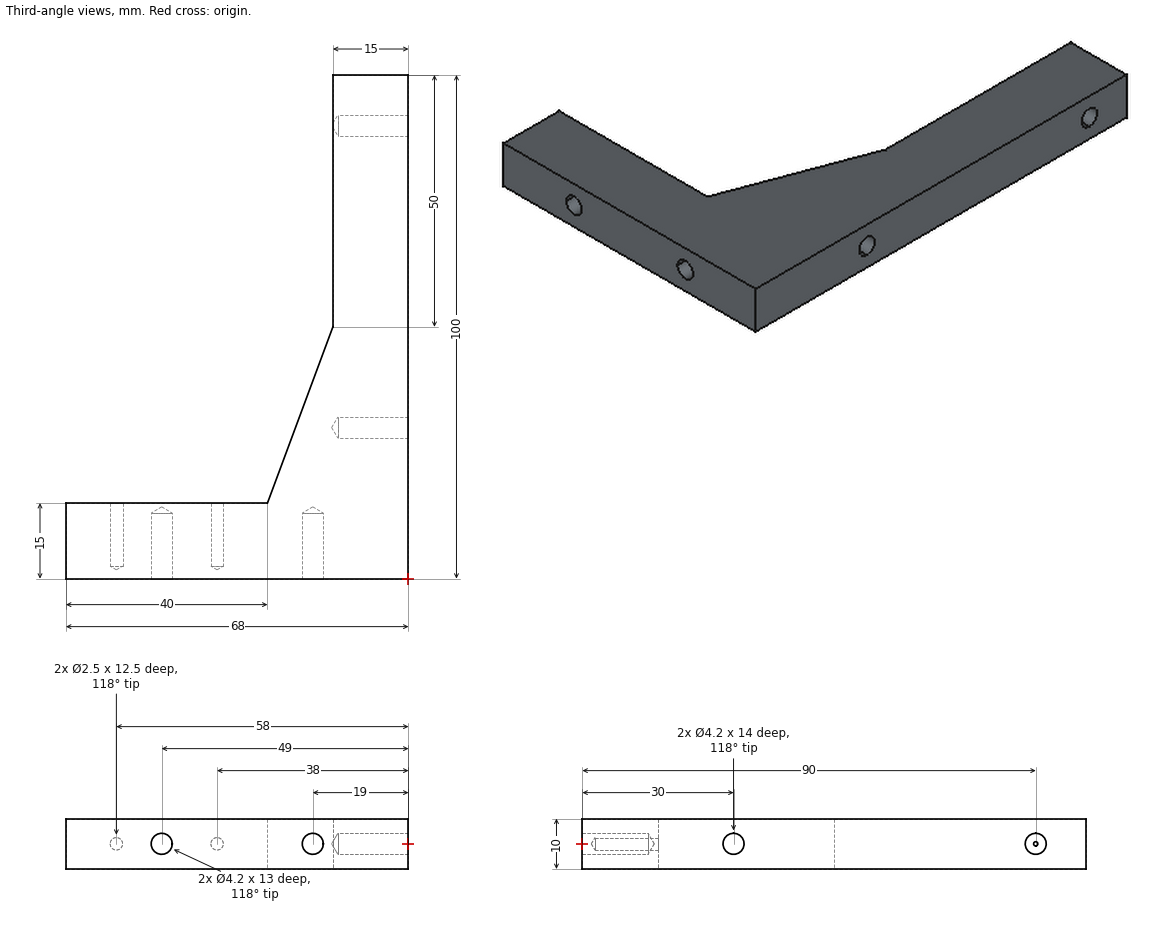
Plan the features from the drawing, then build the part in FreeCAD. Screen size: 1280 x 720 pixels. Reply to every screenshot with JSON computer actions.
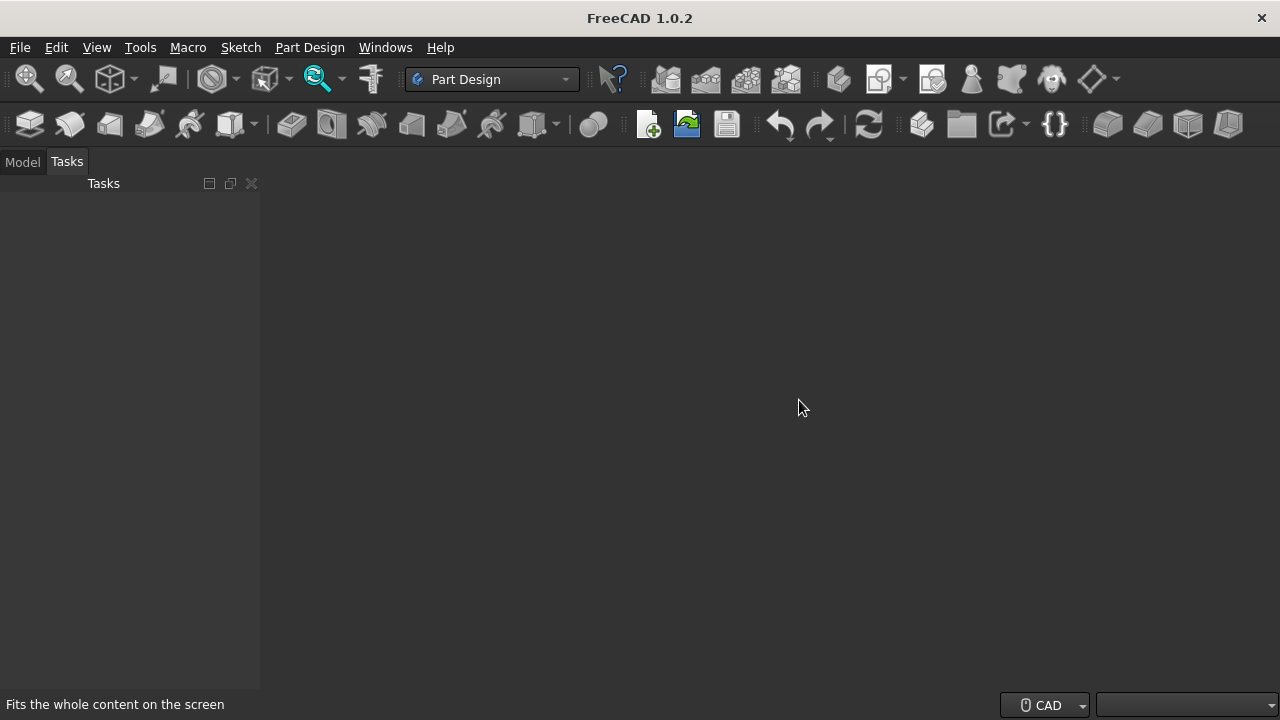
{"action": "key", "text": "ctrl+n"}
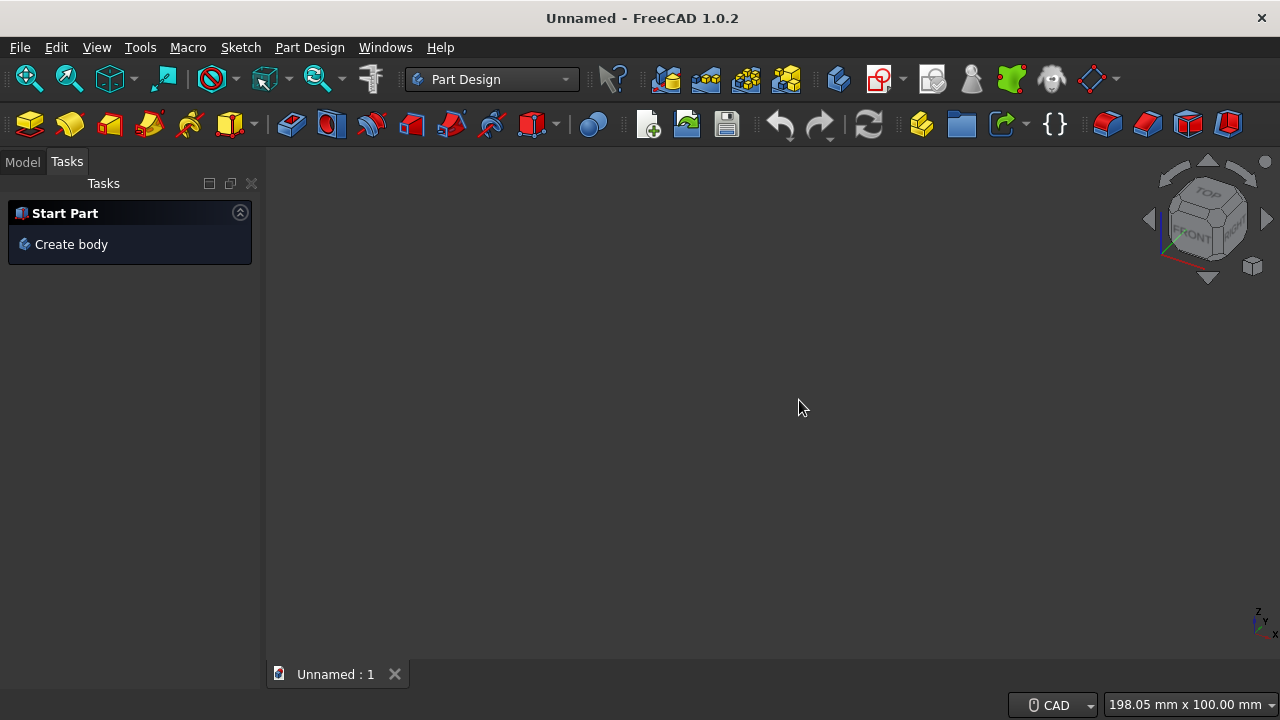
{"action": "left_click", "coordinate": [880, 80]}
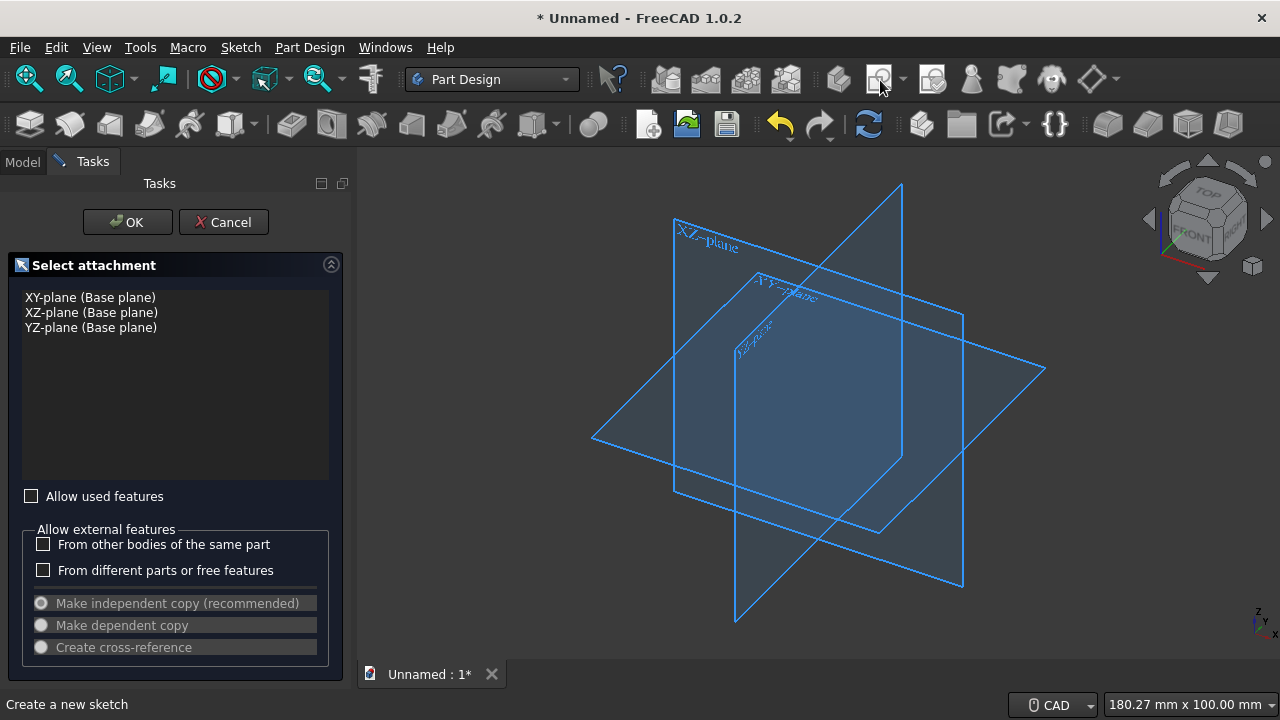
{"action": "left_click", "coordinate": [82, 298]}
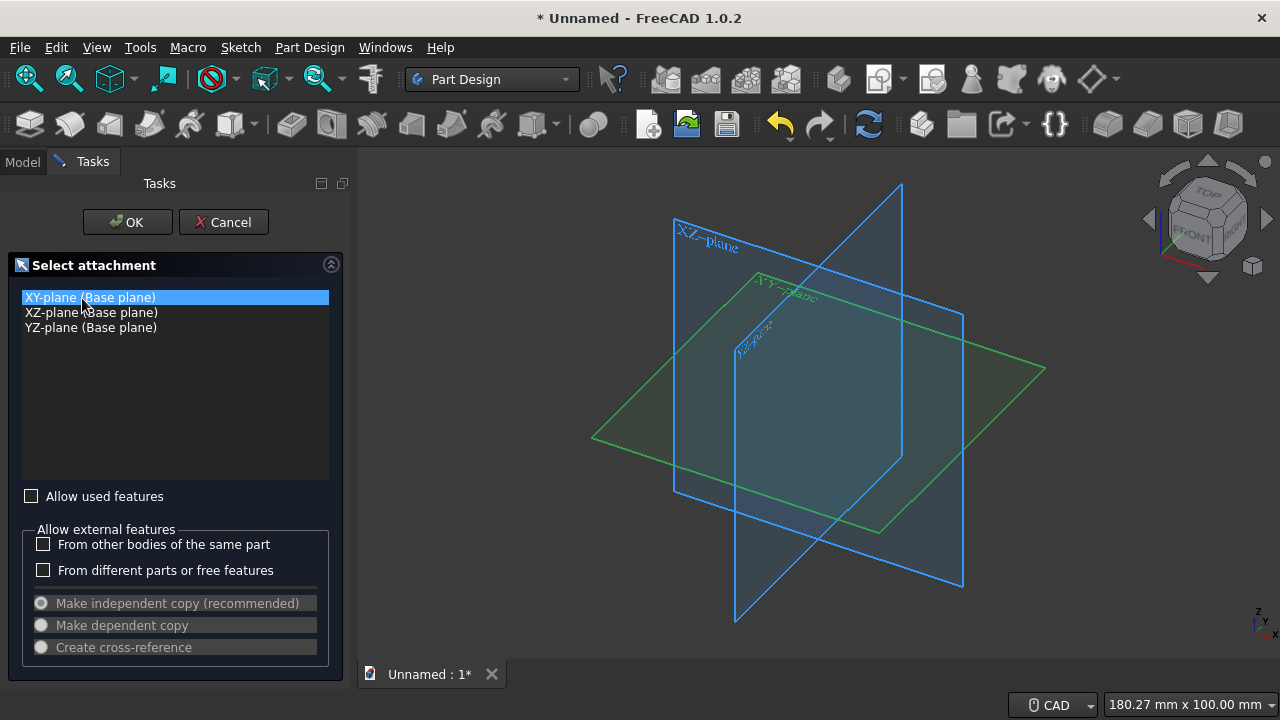
{"action": "left_click", "coordinate": [128, 222]}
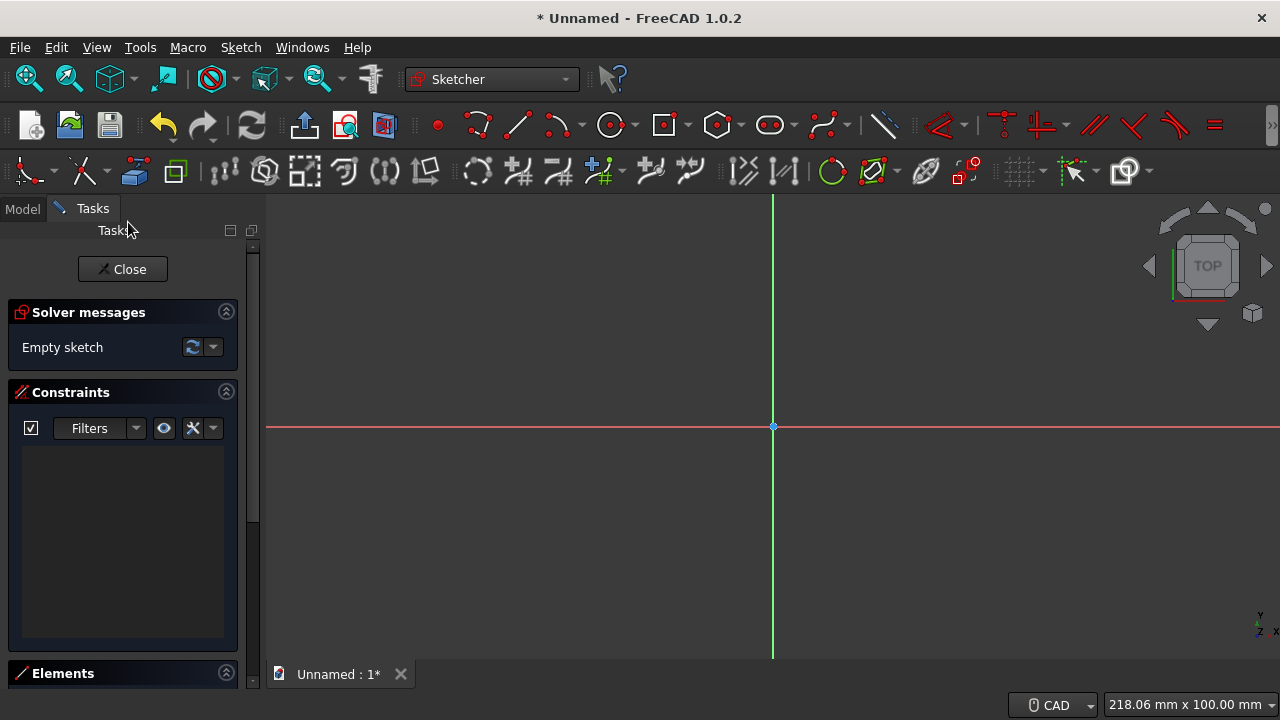
{"action": "scroll", "coordinate": [813, 631], "scroll_direction": "down", "scroll_amount": 3}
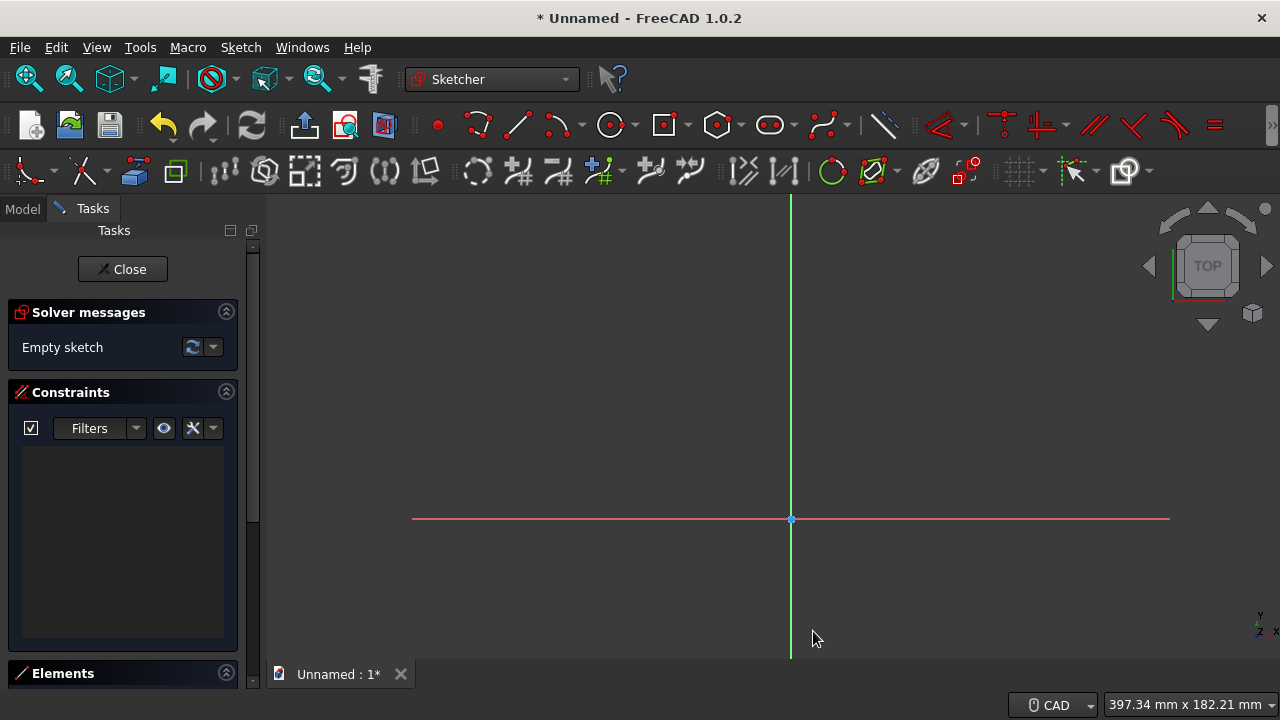
{"action": "key", "text": "g m"}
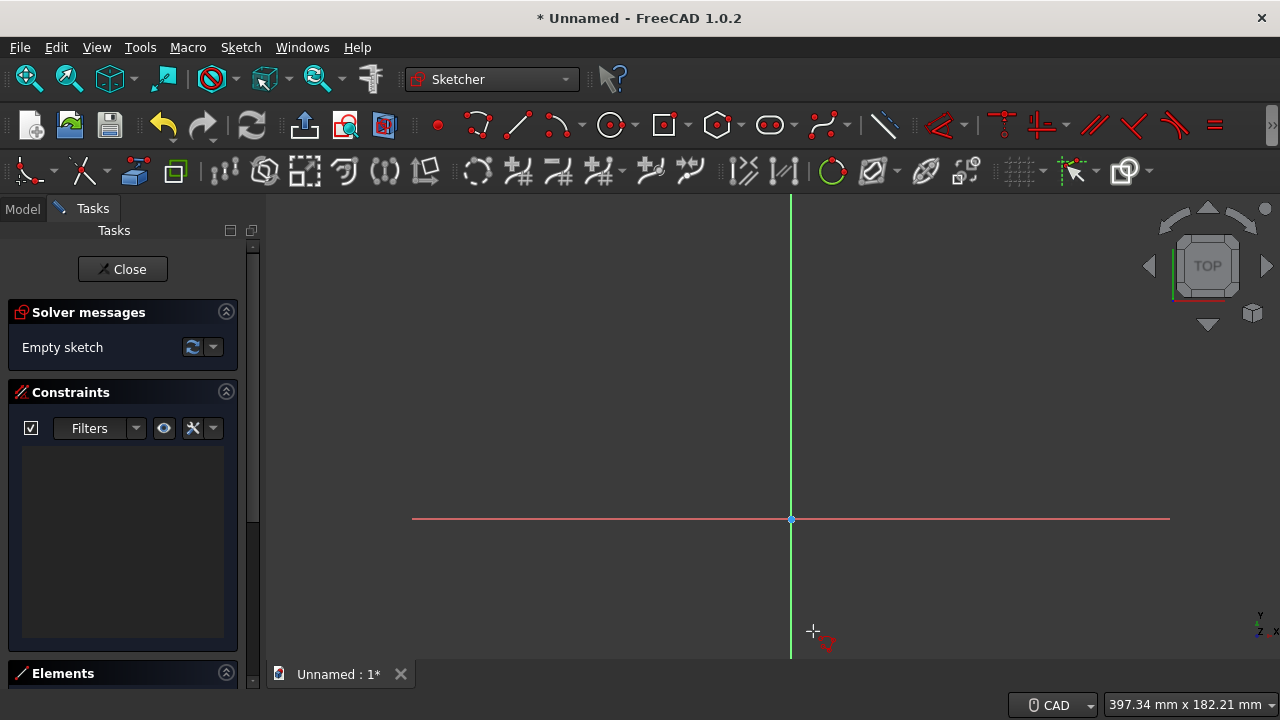
{"action": "left_click", "coordinate": [791, 519]}
{"action": "left_click", "coordinate": [782, 264]}
{"action": "left_click", "coordinate": [753, 264]}
{"action": "left_click", "coordinate": [753, 392]}
{"action": "left_click", "coordinate": [720, 481]}
{"action": "left_click", "coordinate": [618, 481]}
{"action": "left_click", "coordinate": [618, 510]}
{"action": "left_click", "coordinate": [791, 519]}
{"action": "key", "text": "Escape"}
{"action": "key", "text": "Escape"}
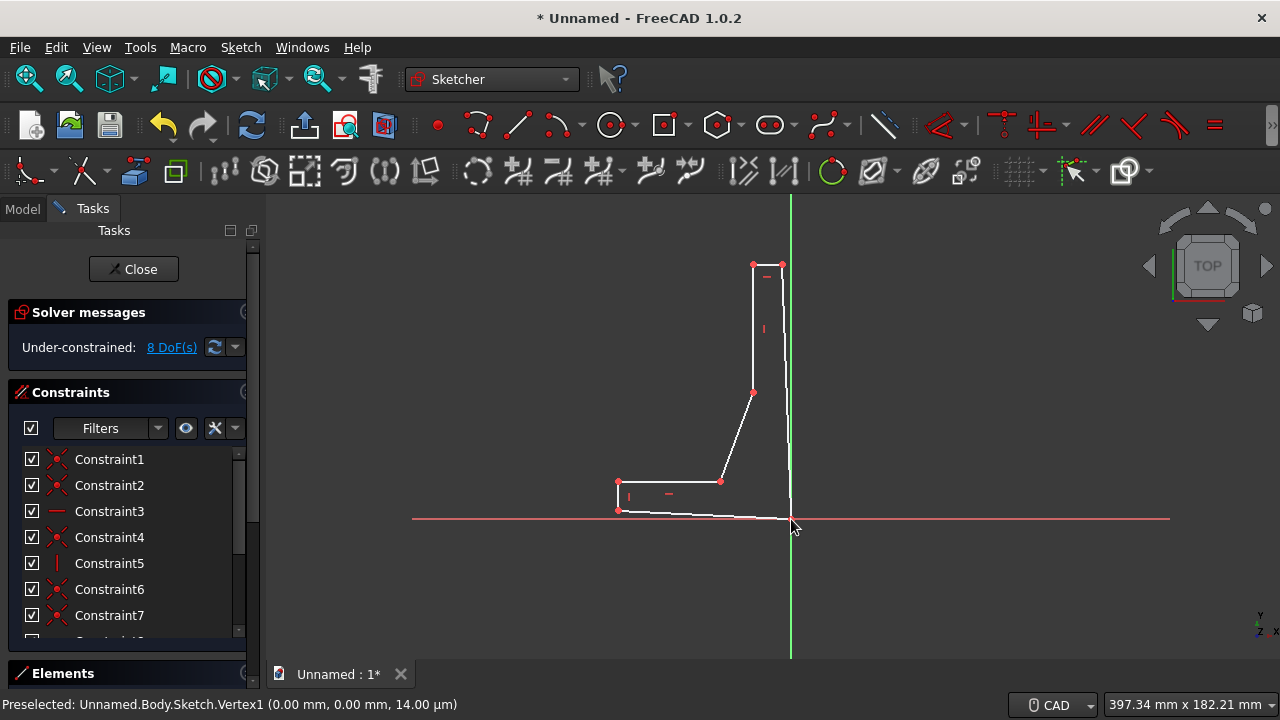
{"action": "left_click", "coordinate": [789, 443]}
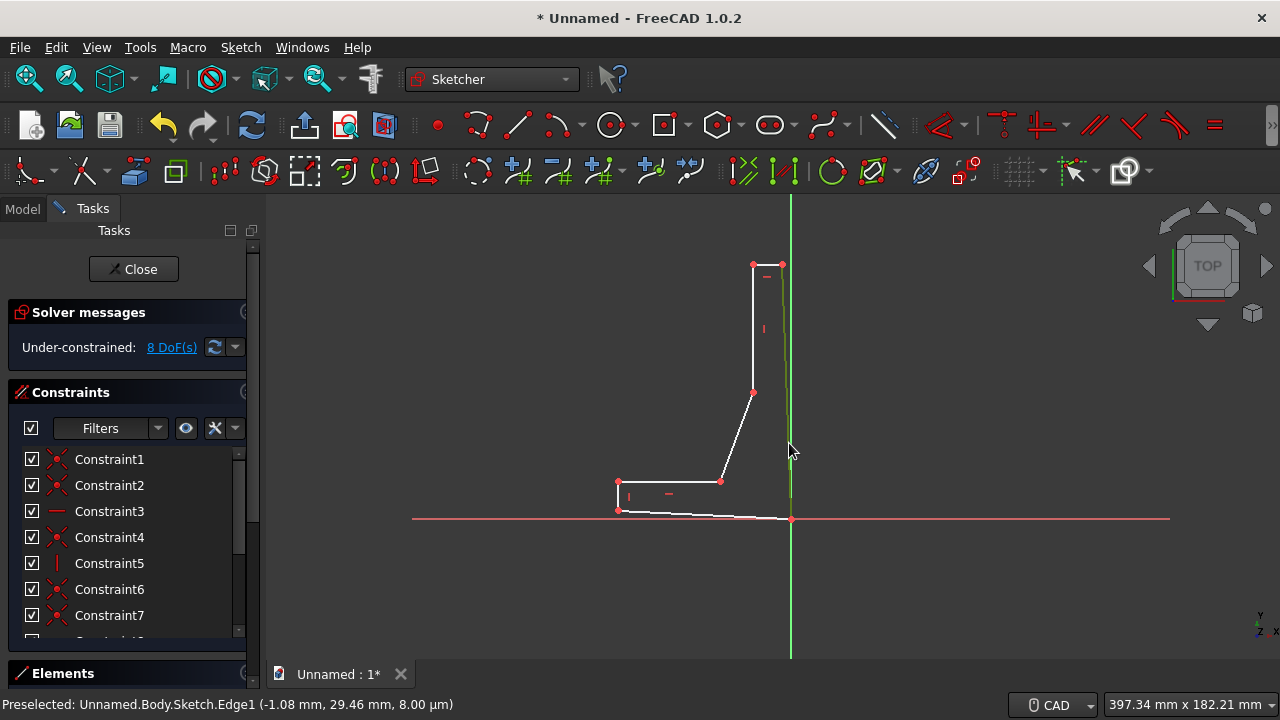
{"action": "key", "text": "v"}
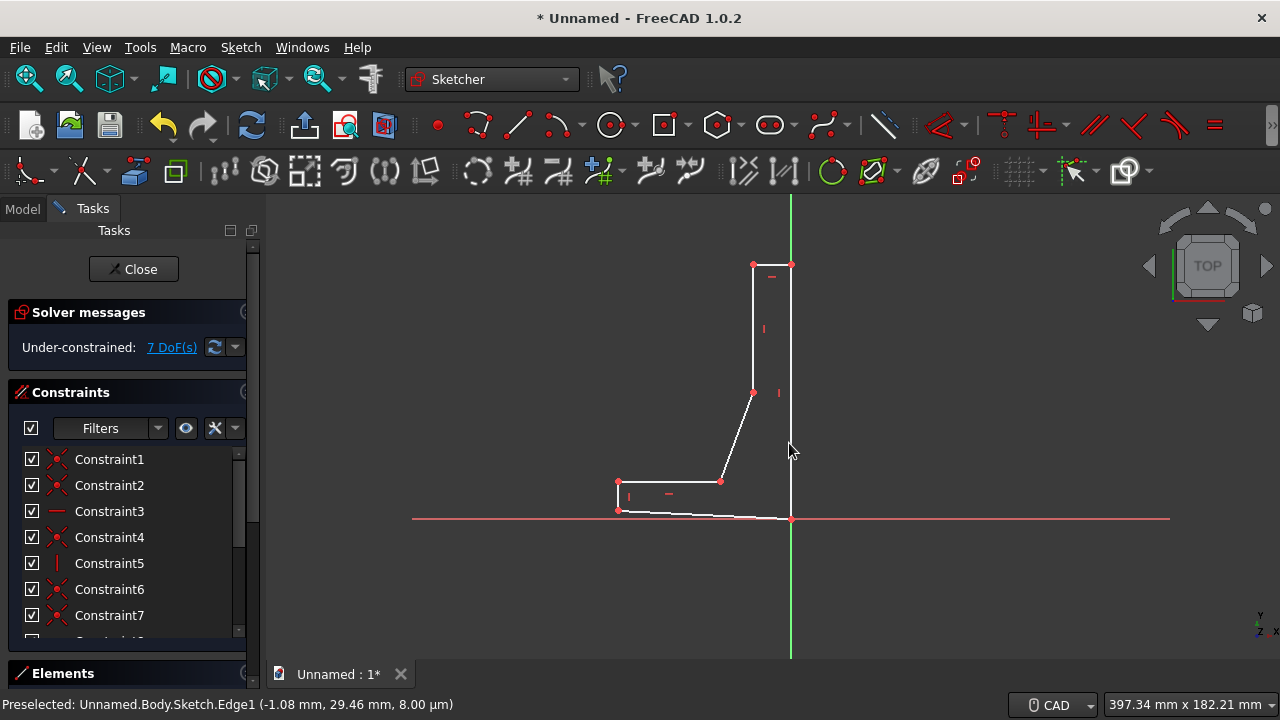
{"action": "left_click", "coordinate": [739, 517]}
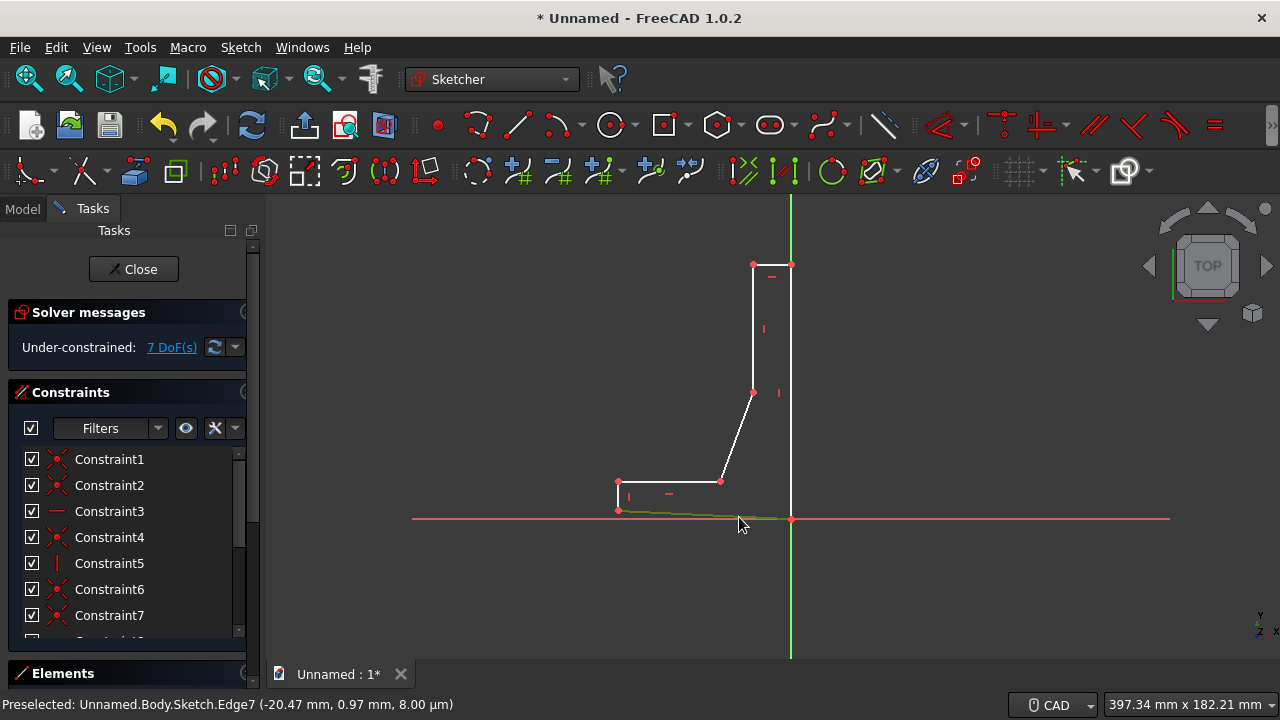
{"action": "left_click", "coordinate": [1068, 126]}